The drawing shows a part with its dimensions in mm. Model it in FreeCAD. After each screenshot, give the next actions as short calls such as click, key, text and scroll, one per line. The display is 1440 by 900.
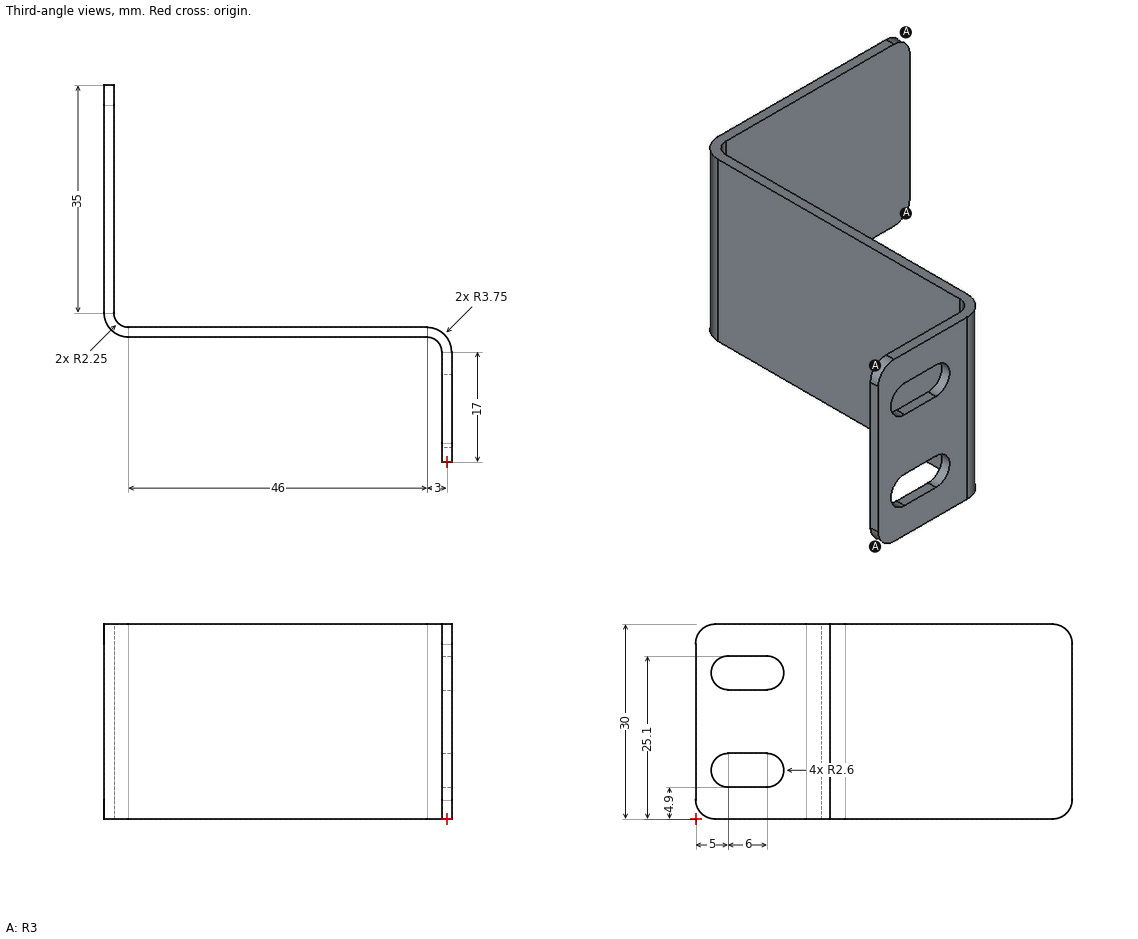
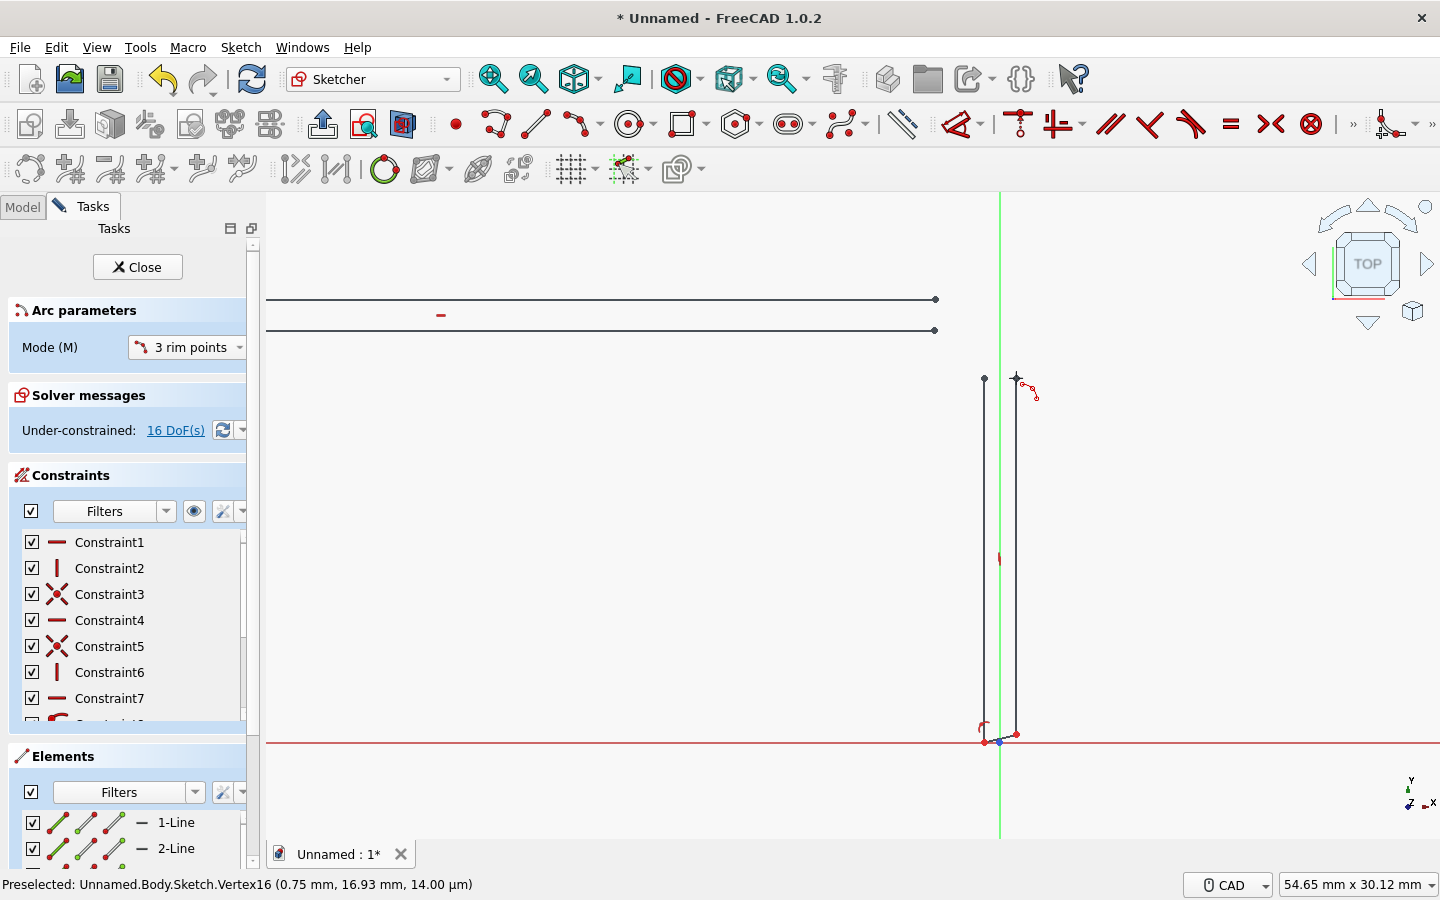
scroll(984, 746, down, 5)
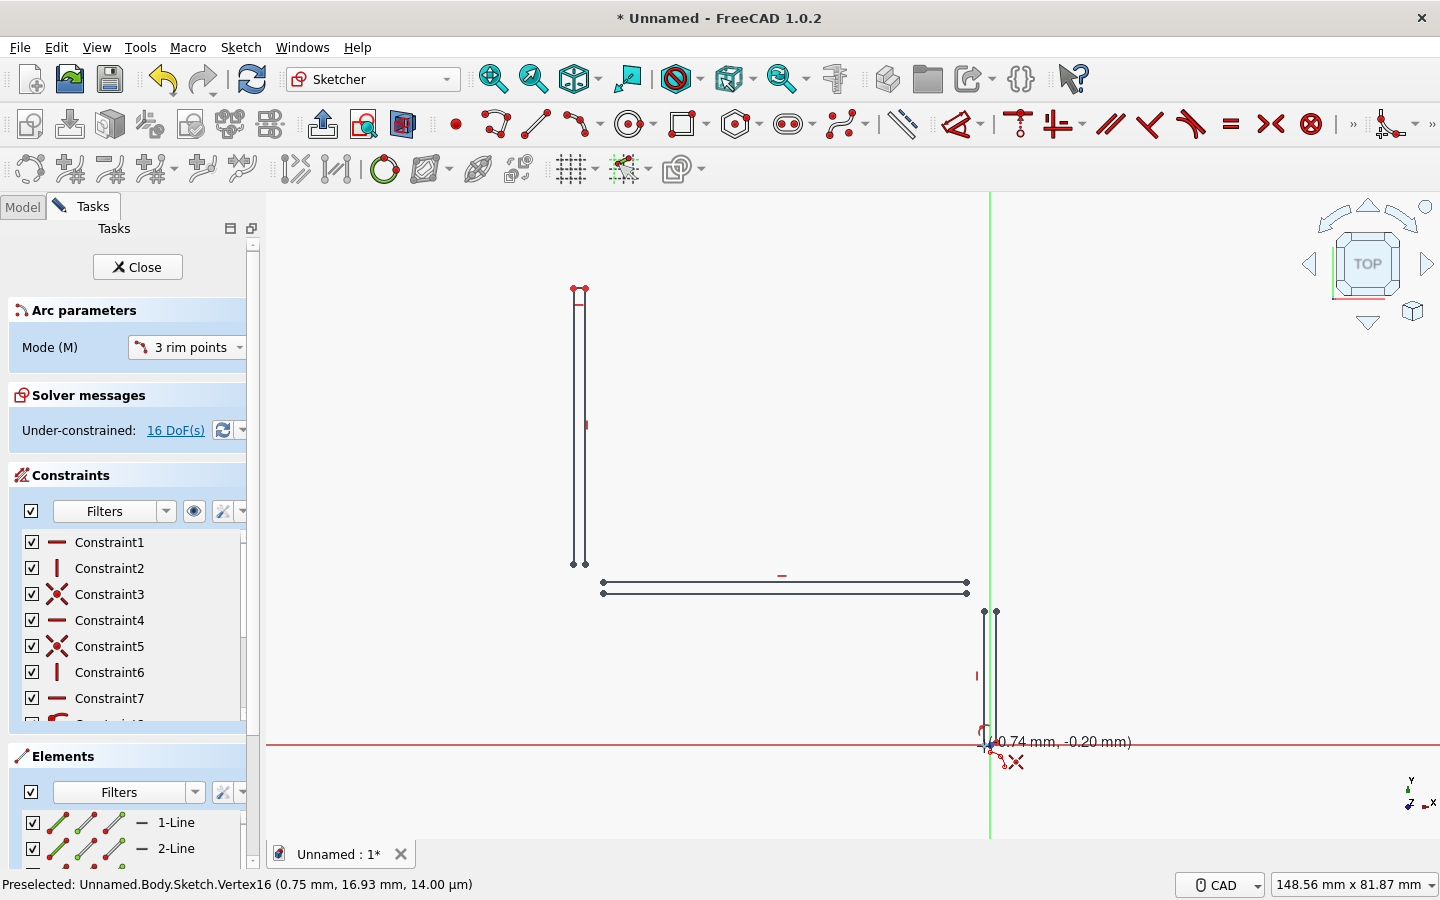
scroll(603, 581, up, 2)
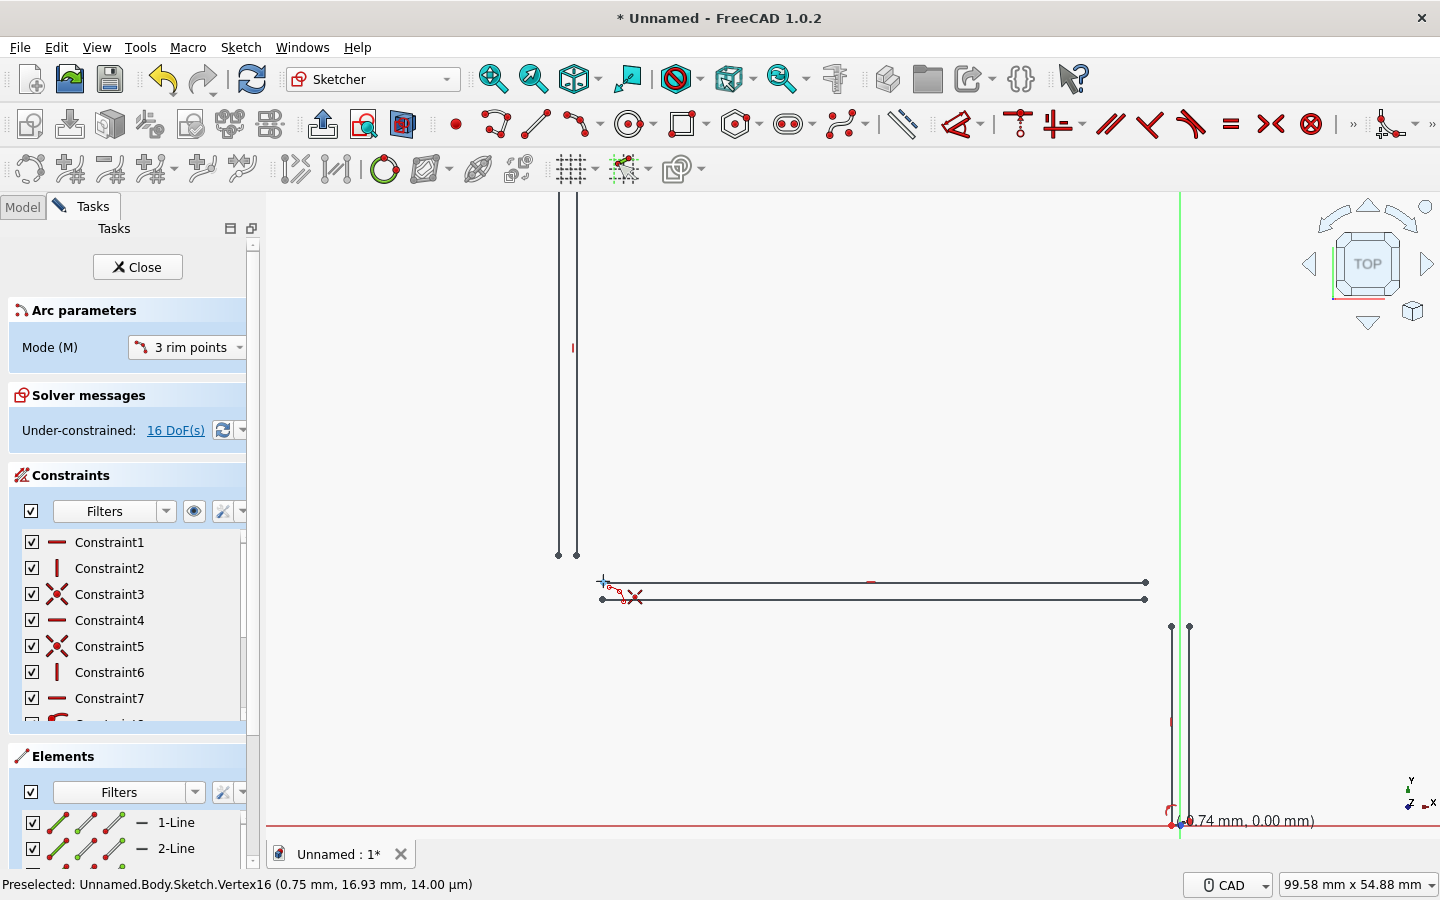
click(604, 583)
click(577, 556)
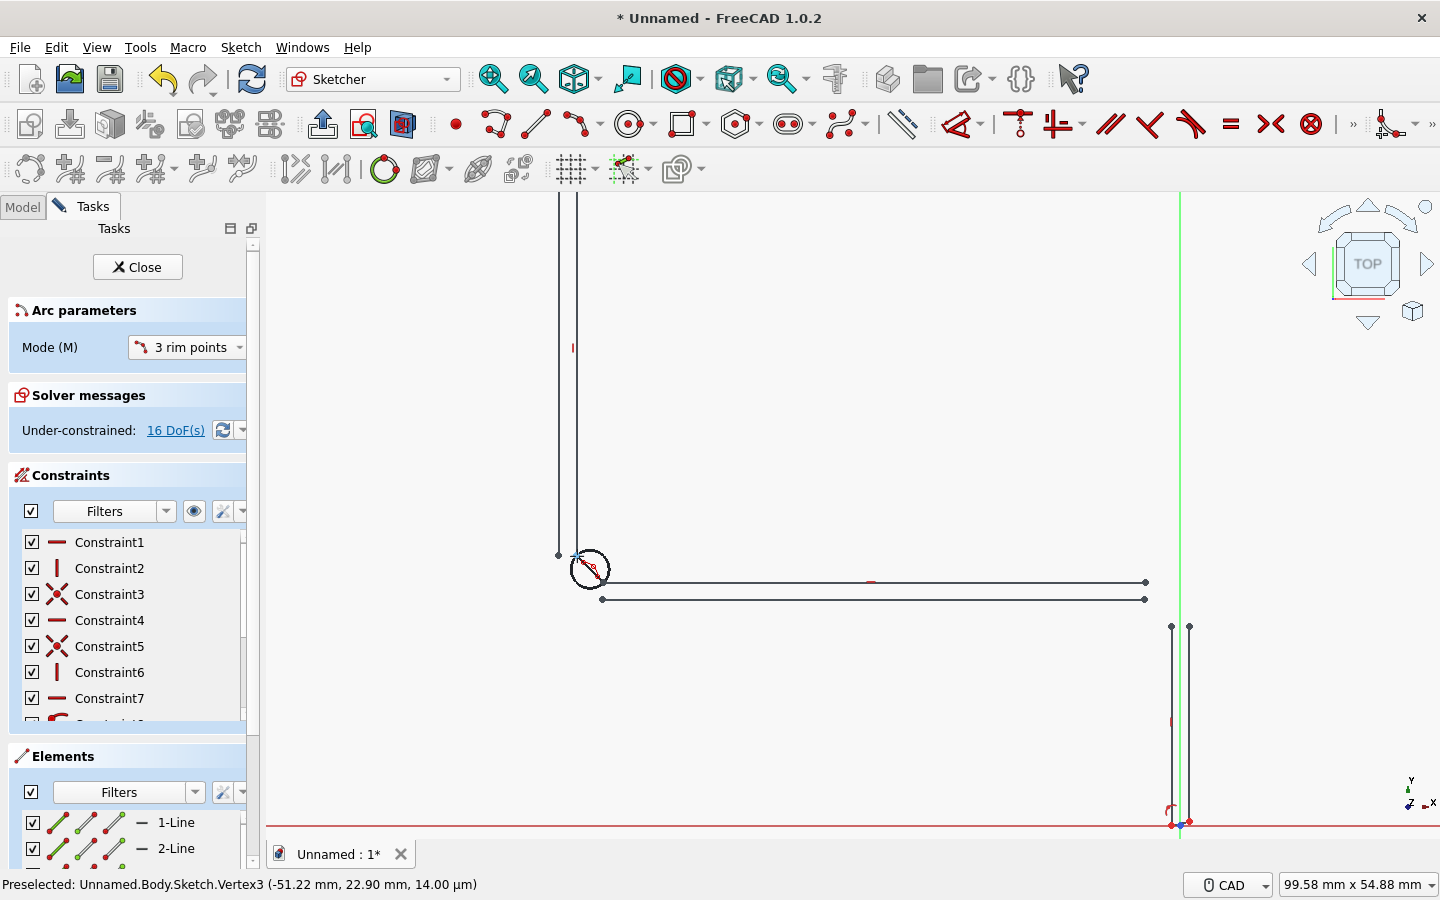
scroll(584, 573, up, 4)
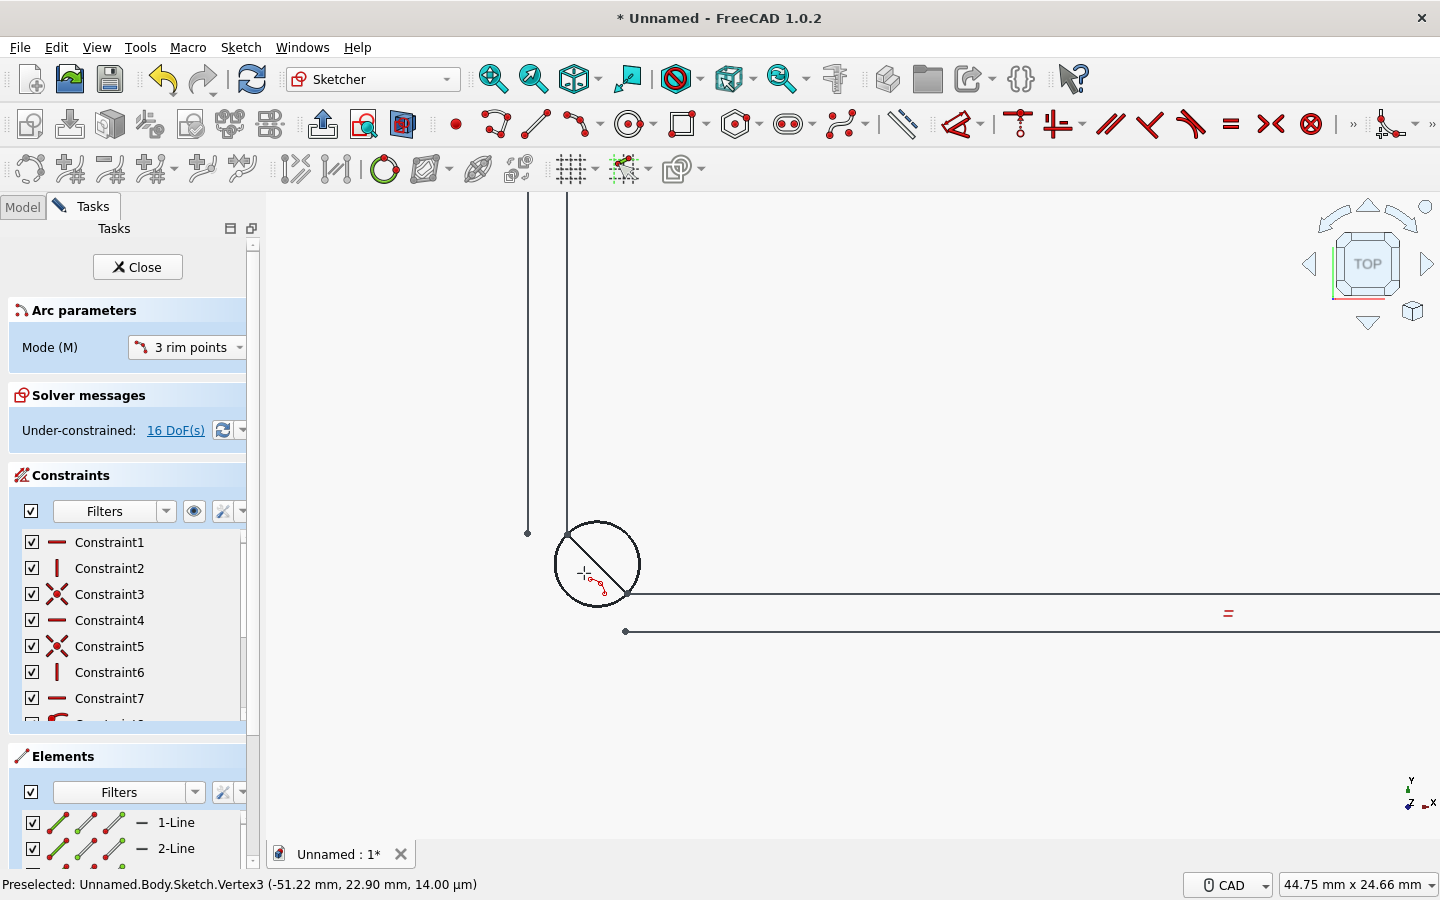
click(584, 573)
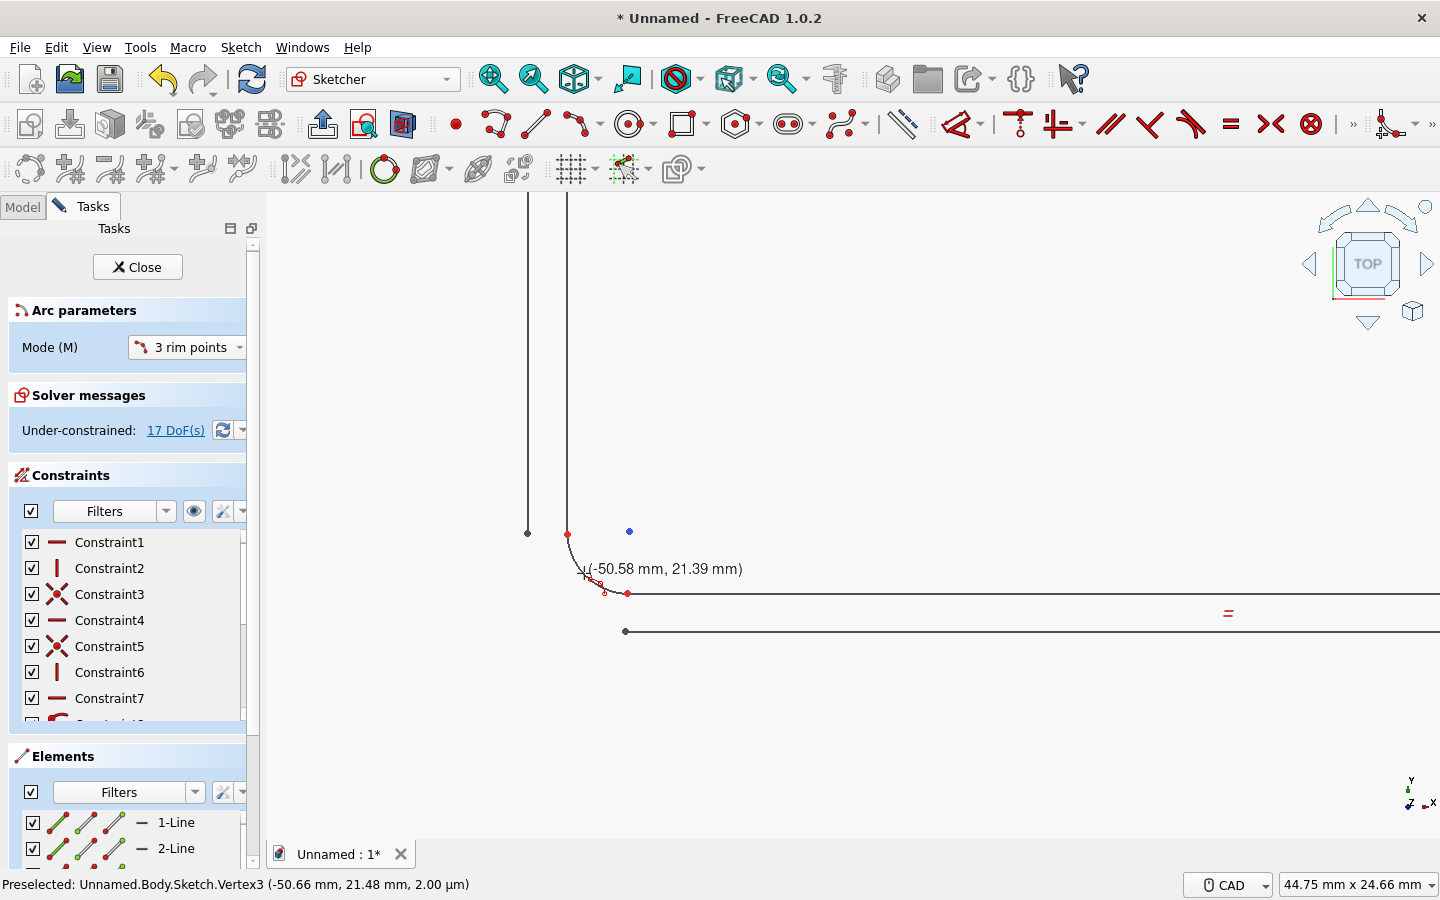
click(528, 534)
click(626, 632)
click(556, 601)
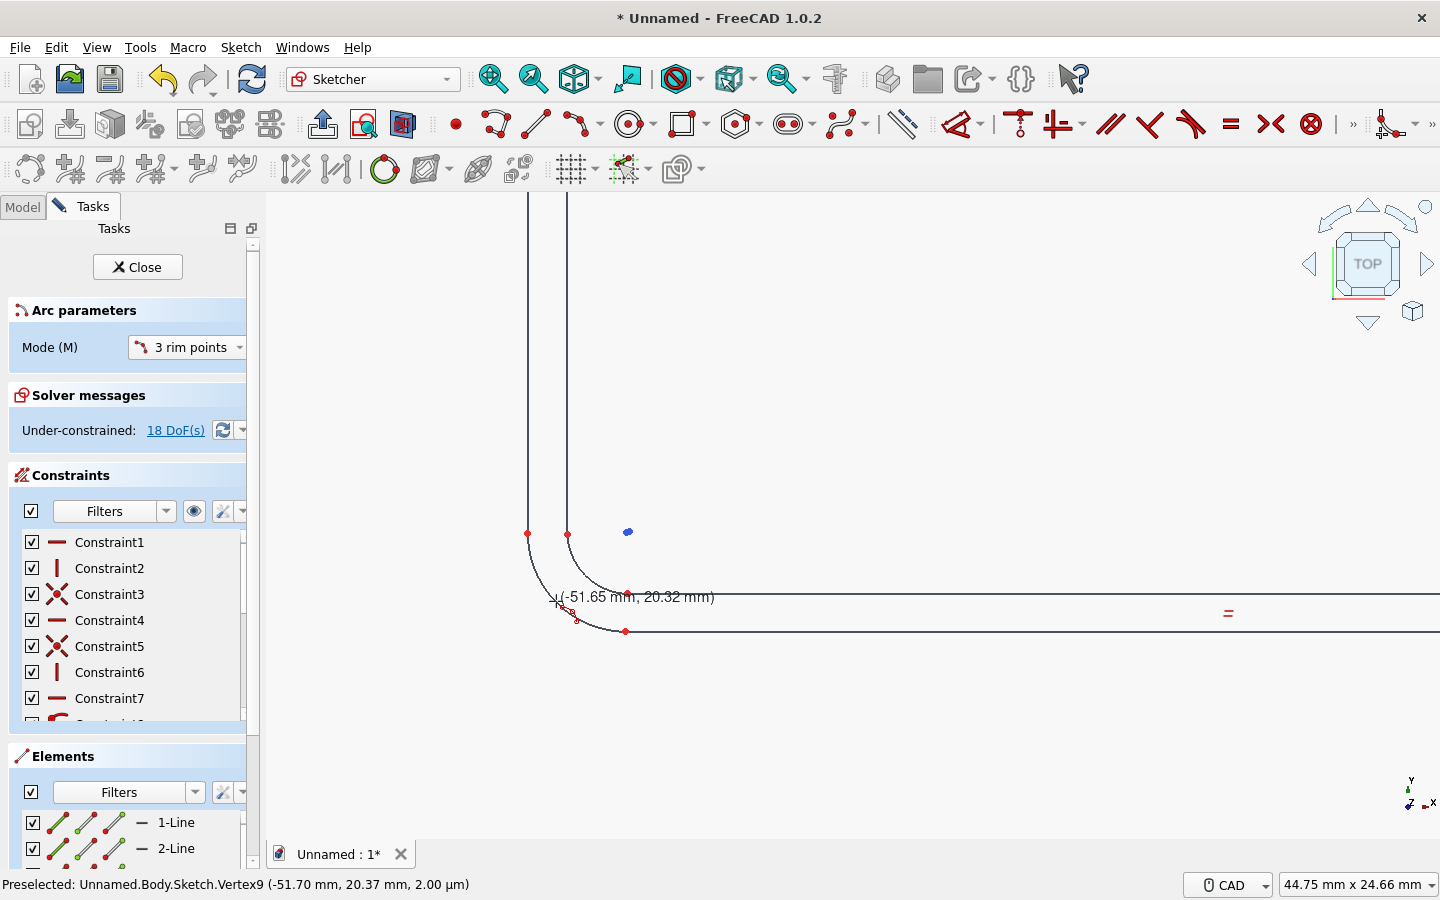
scroll(593, 576, down, 6)